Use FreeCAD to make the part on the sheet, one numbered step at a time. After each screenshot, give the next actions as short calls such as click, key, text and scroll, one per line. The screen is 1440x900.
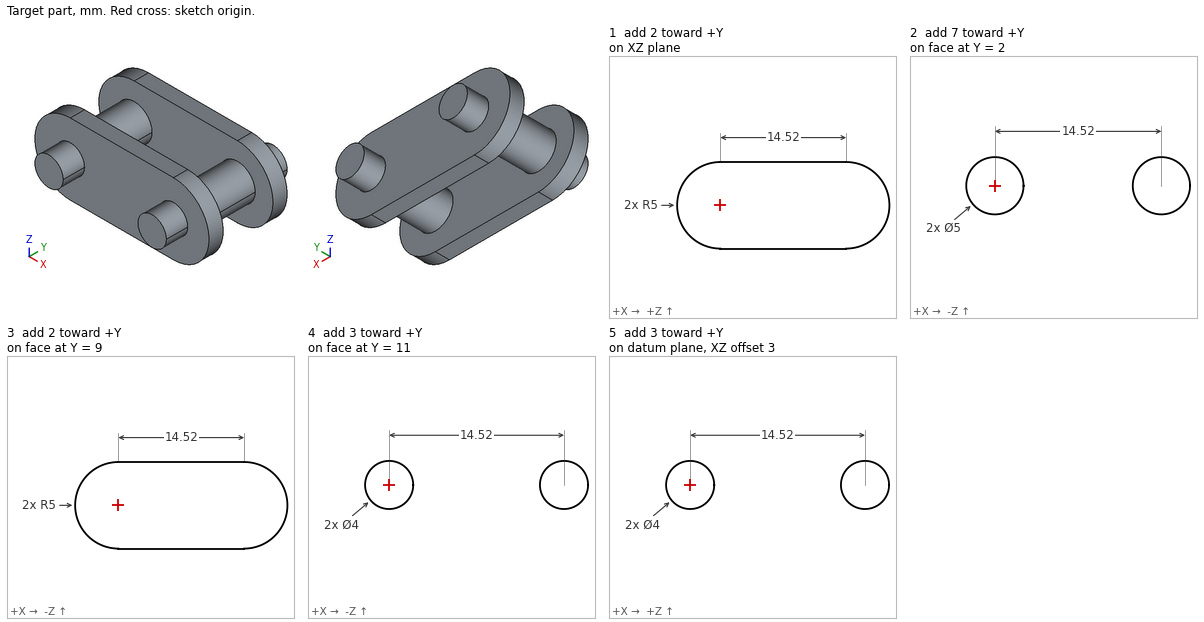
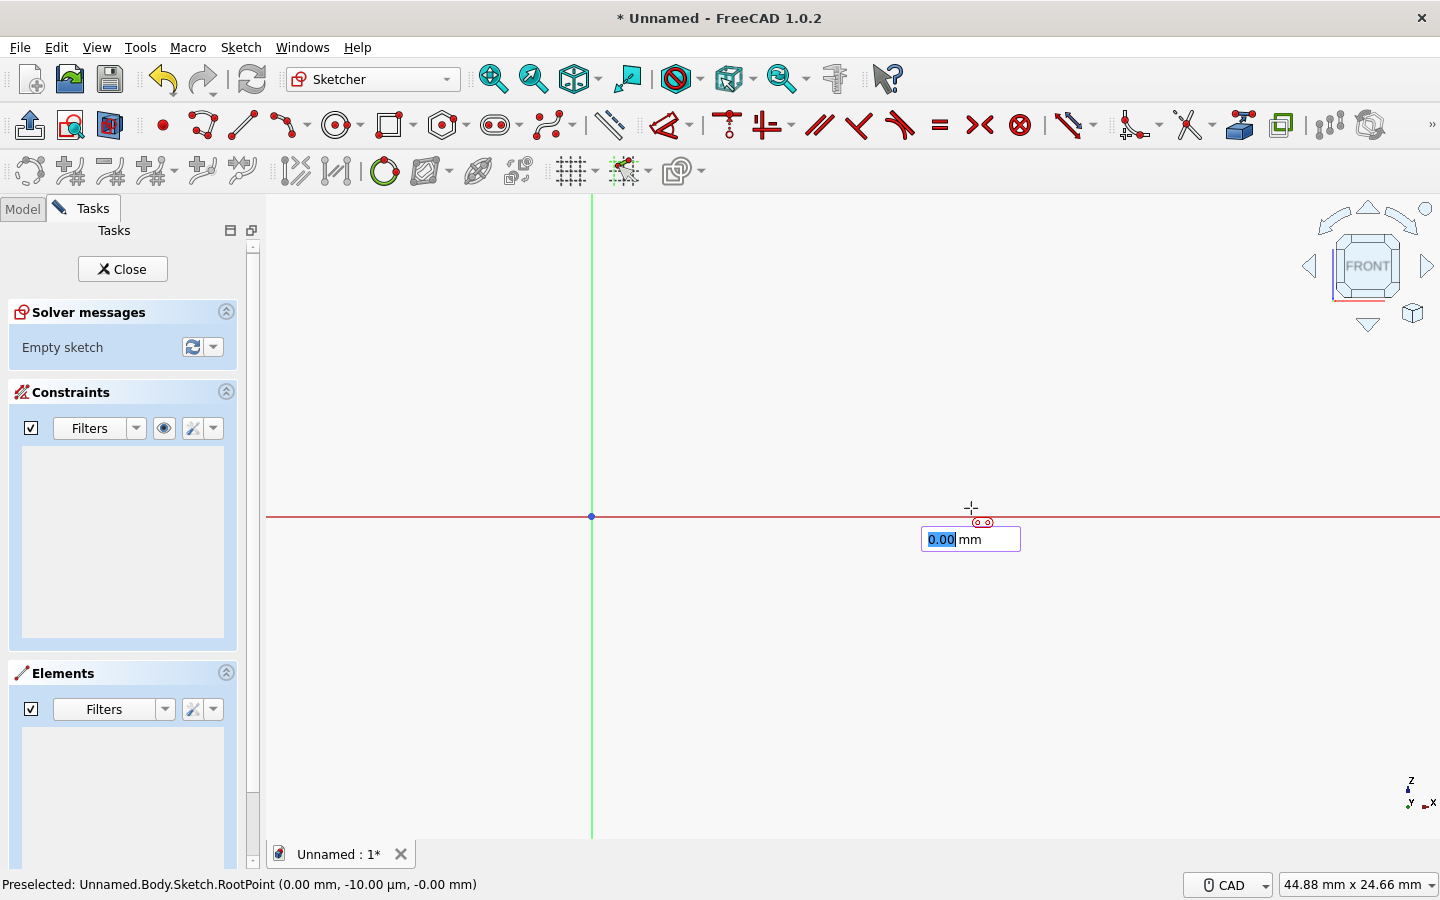
click(781, 647)
key(Escape)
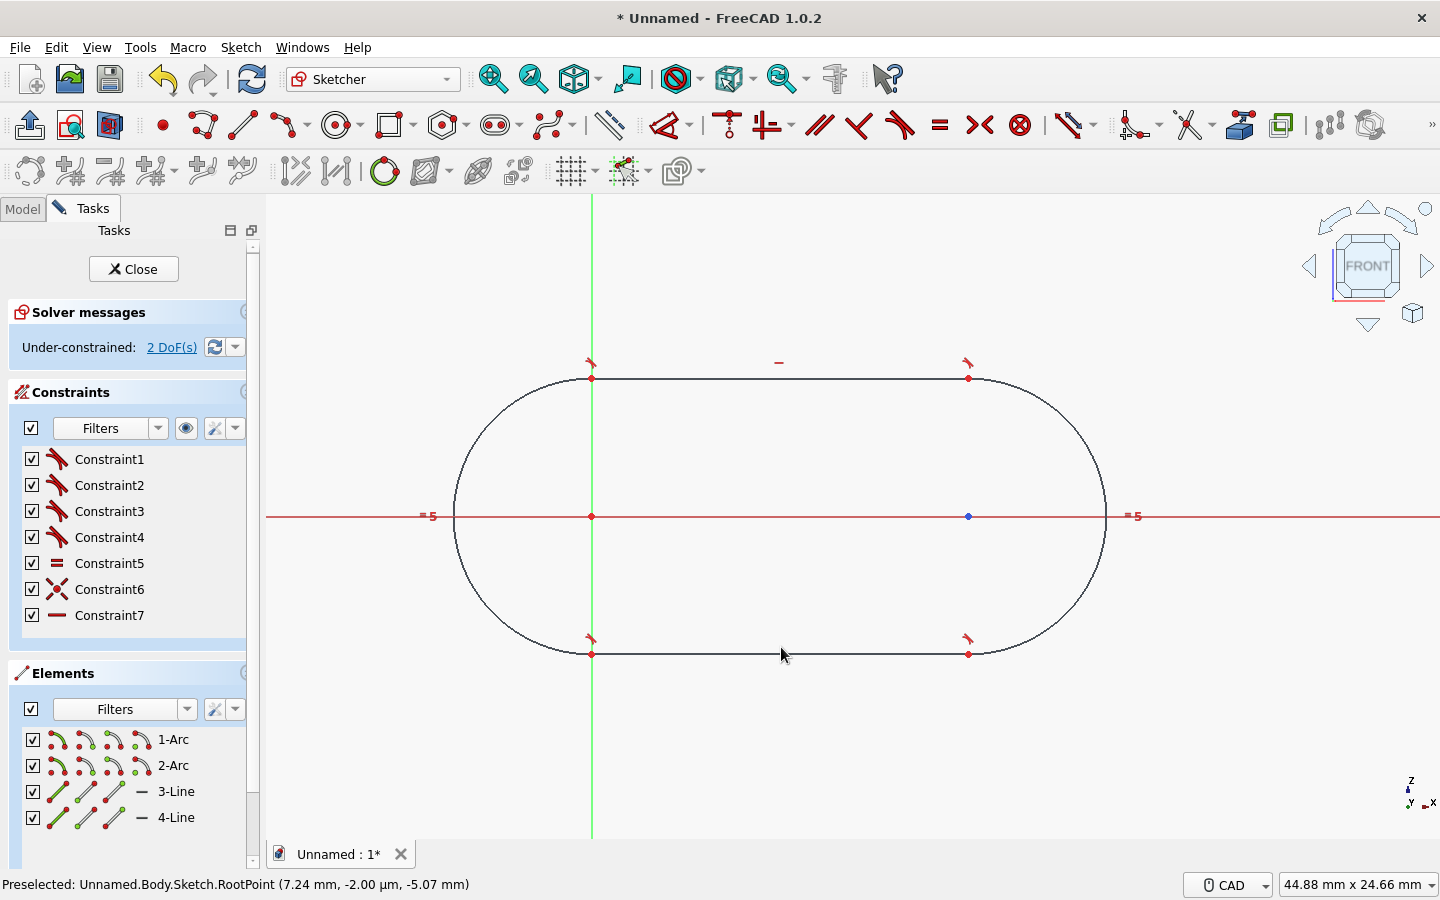
click(664, 126)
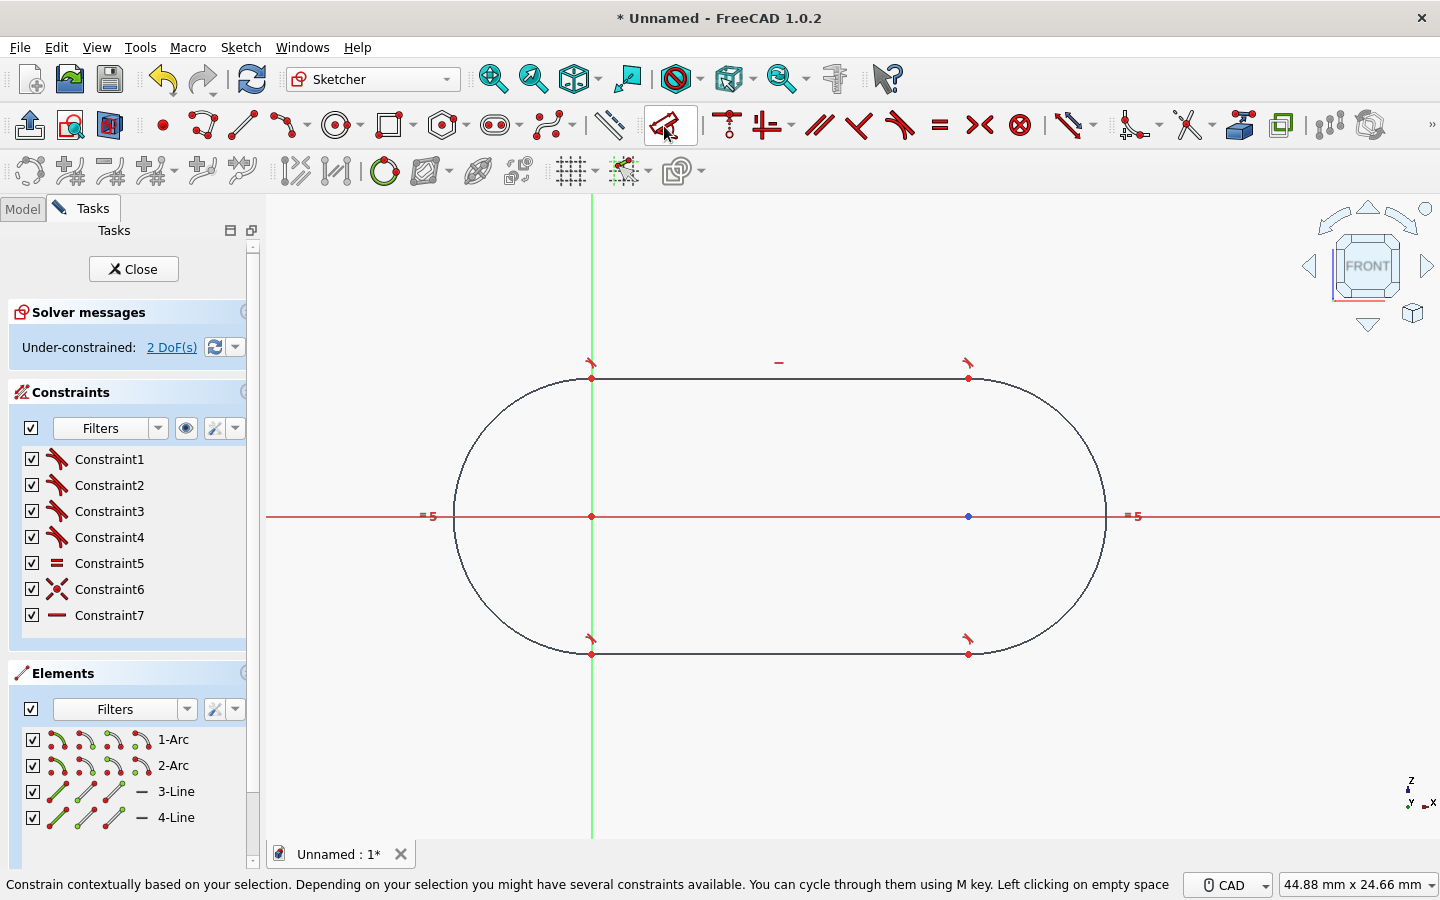
click(480, 435)
click(454, 416)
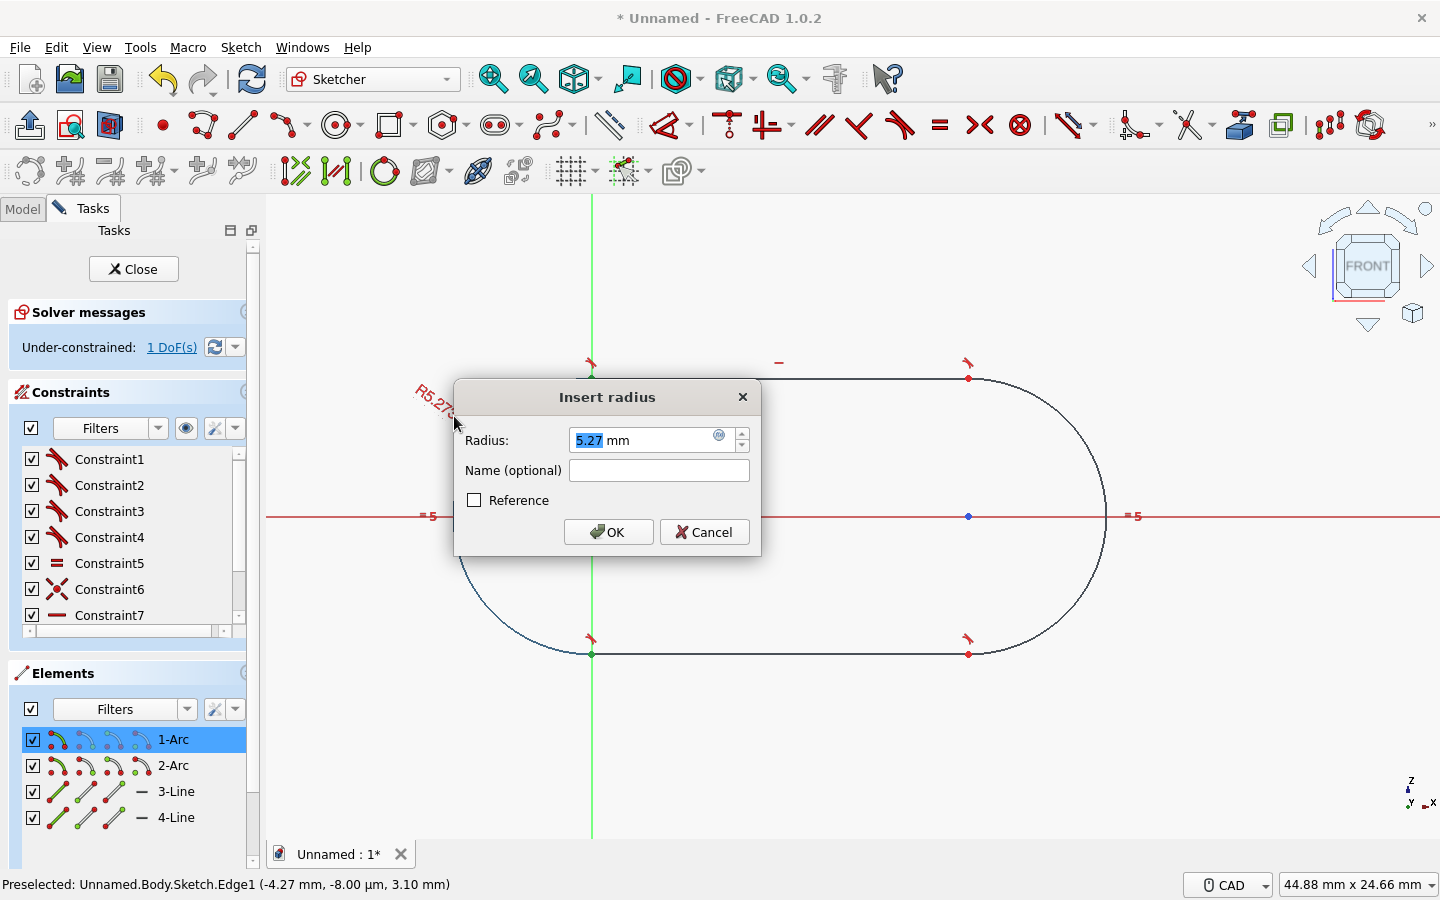
text(5)
key(Return)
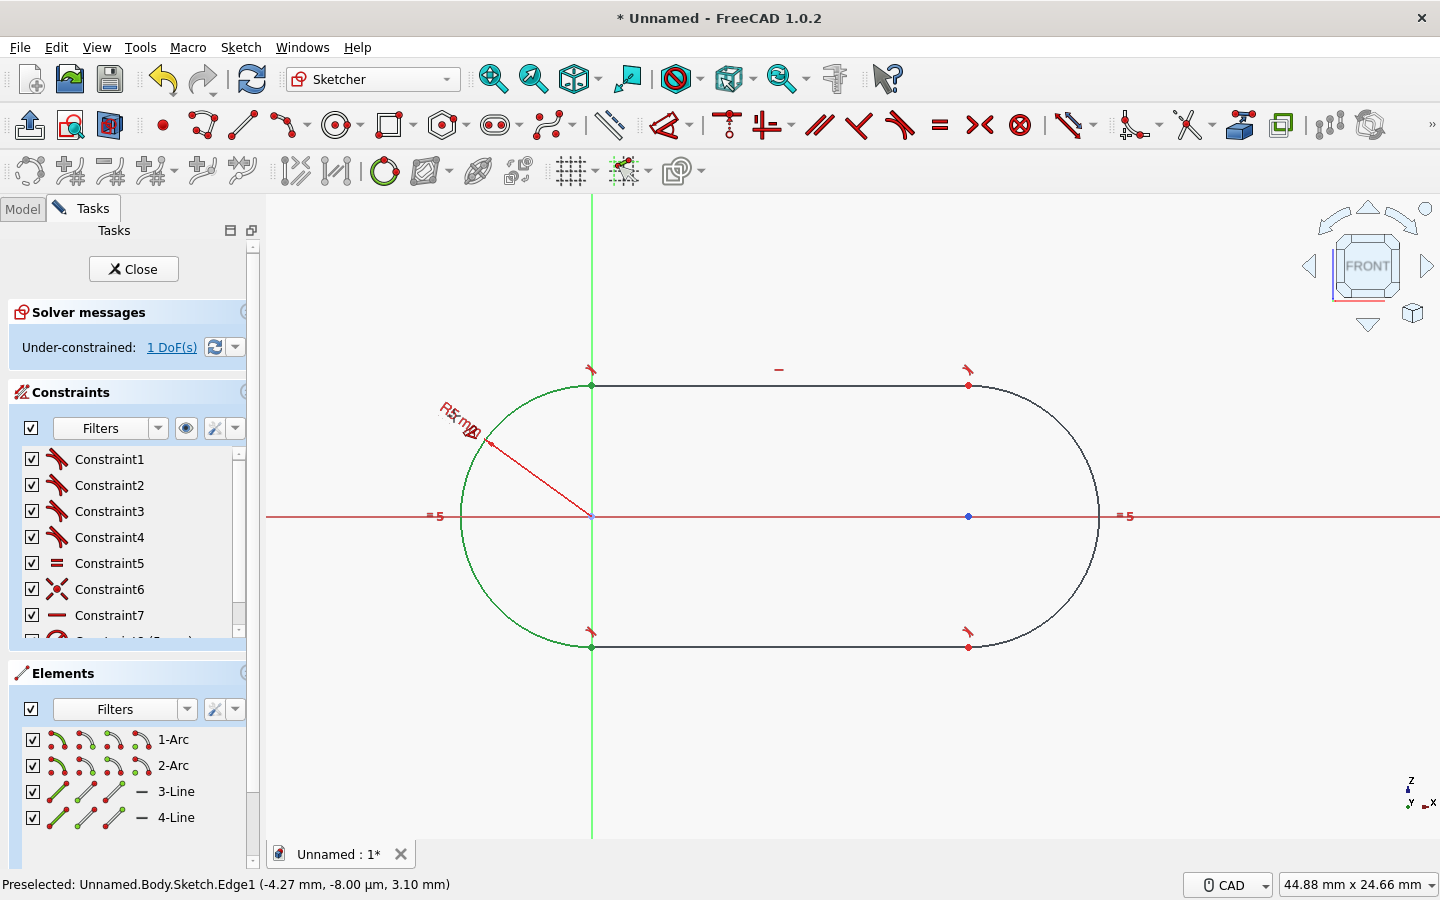
click(705, 386)
click(780, 352)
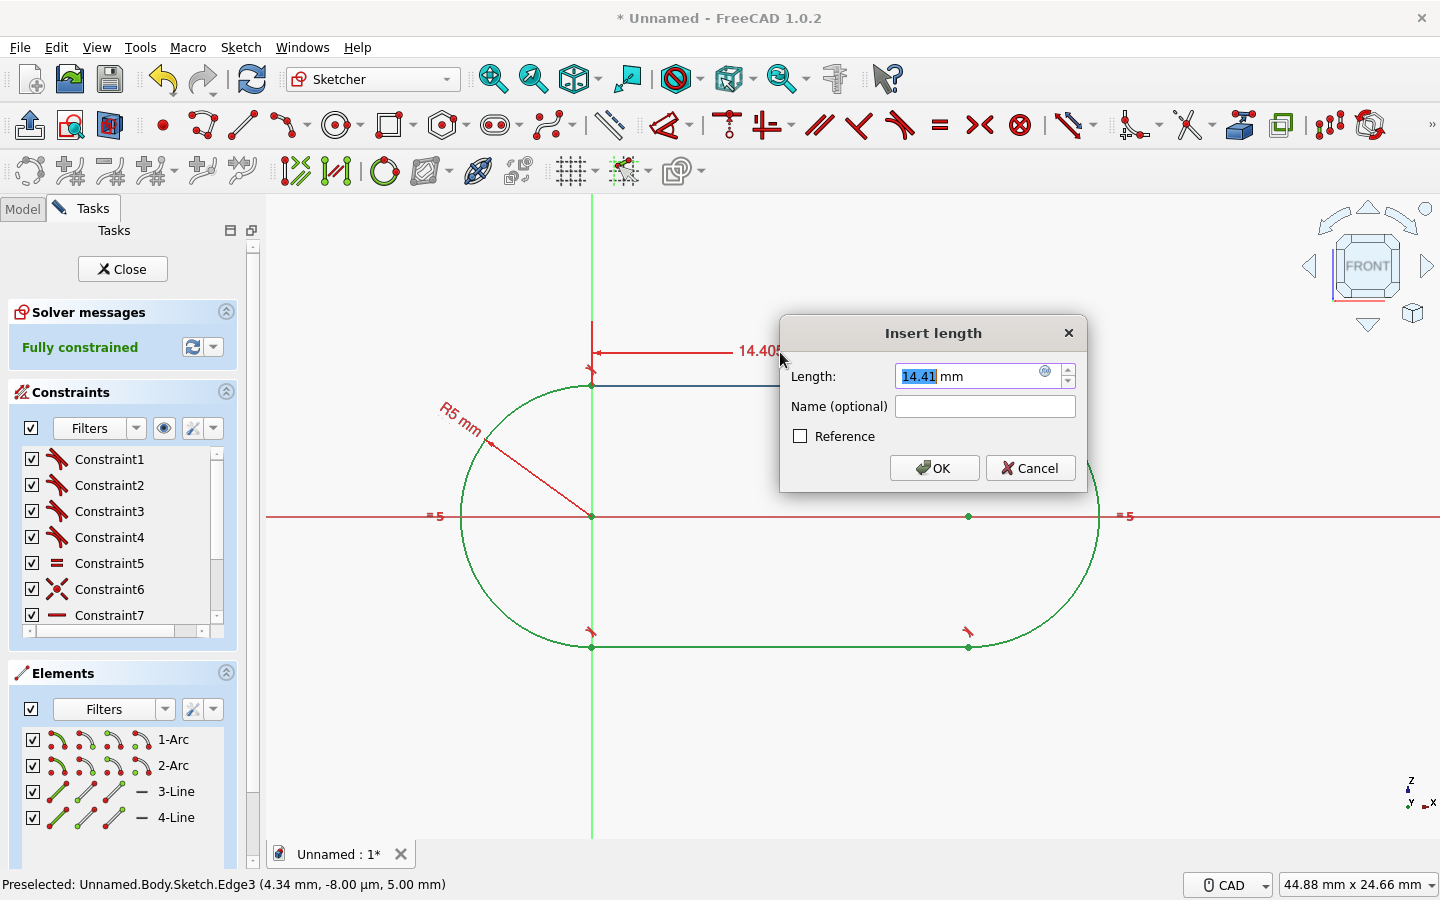
text(14.52)
key(Return)
key(Escape)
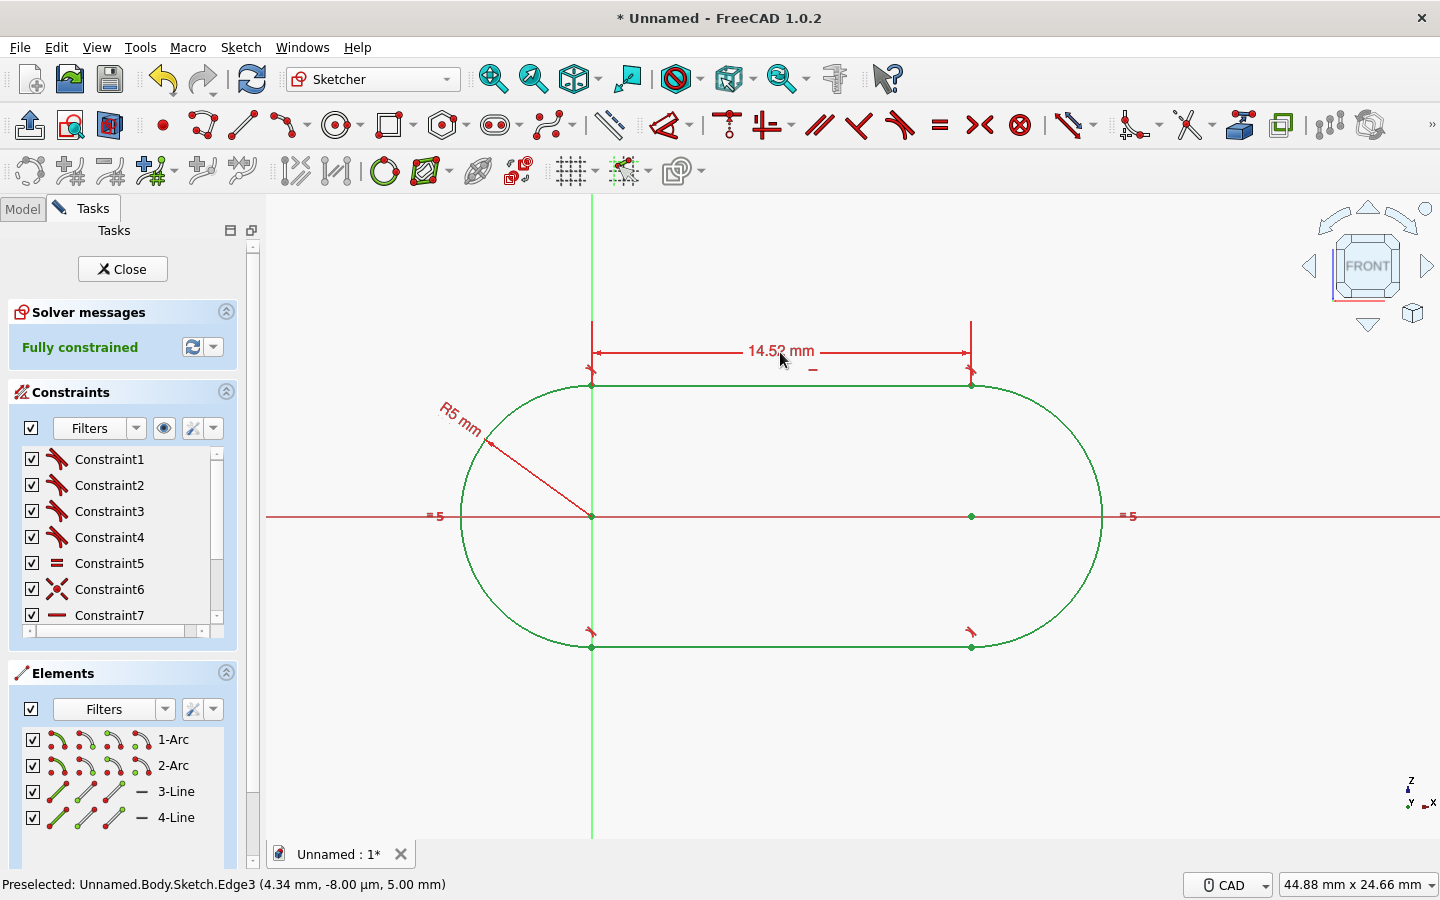
click(123, 269)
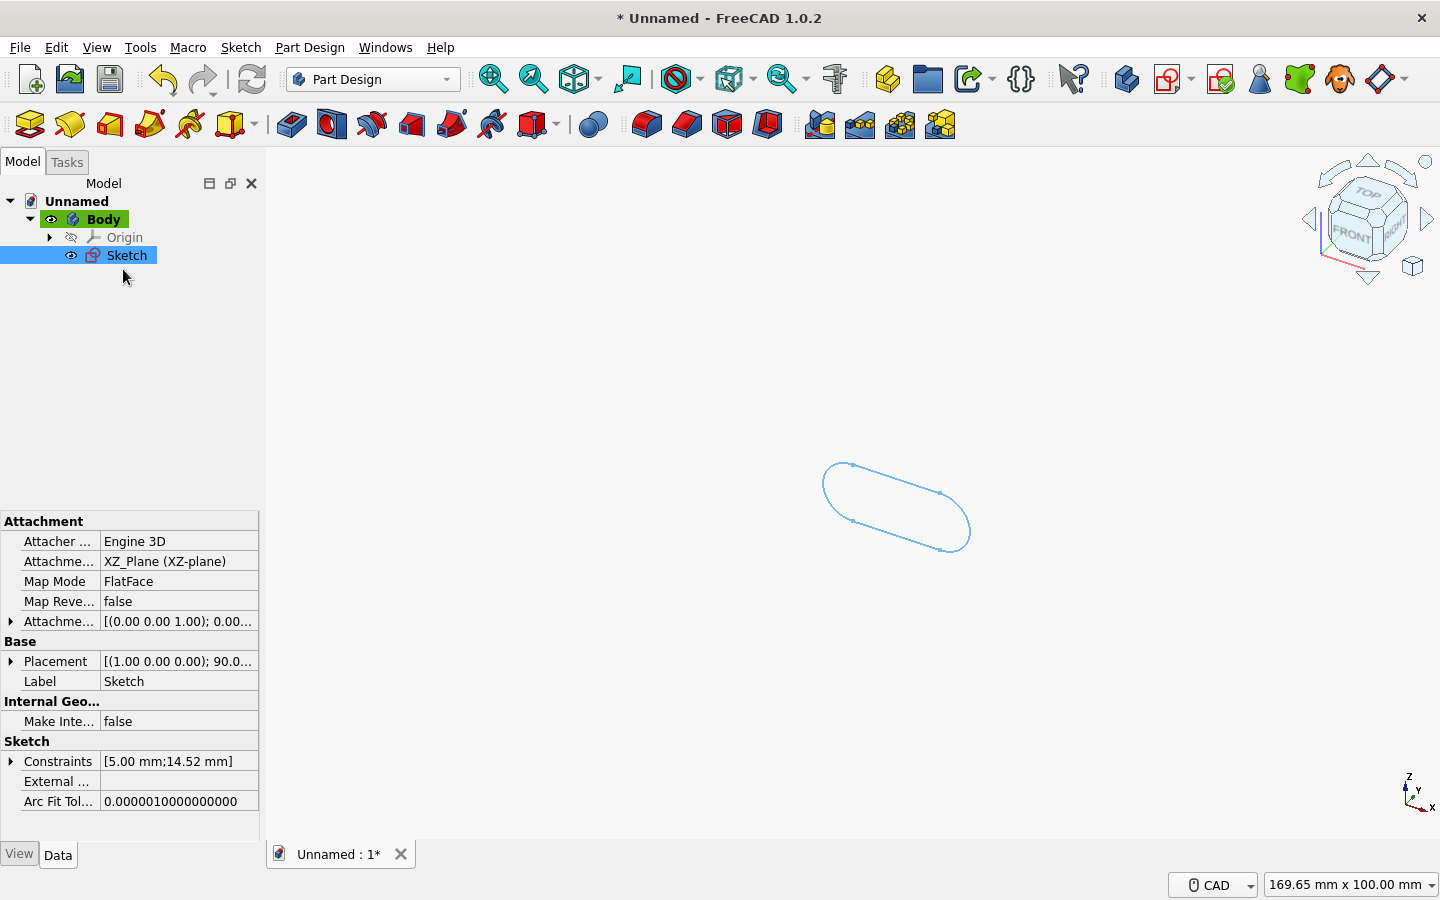
click(30, 124)